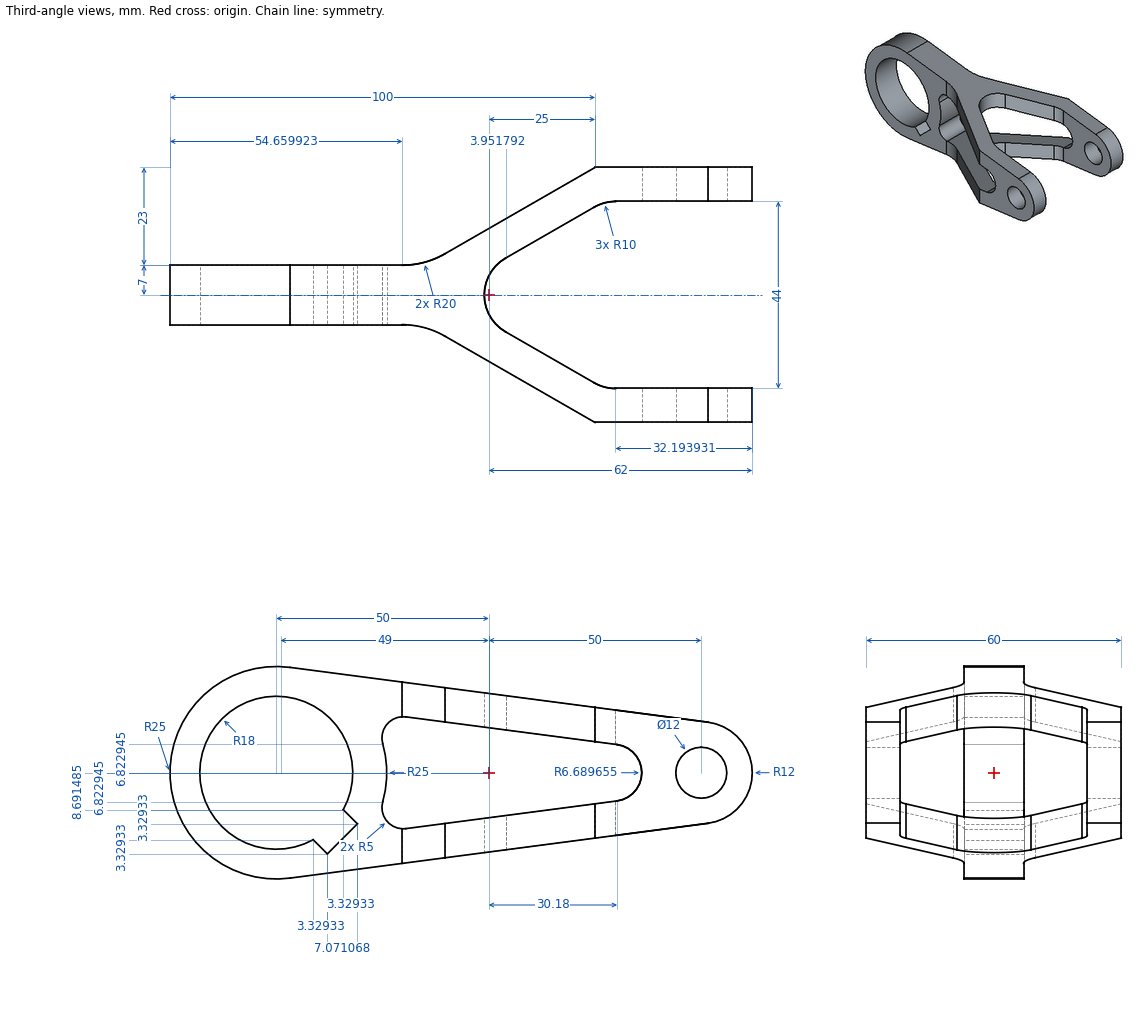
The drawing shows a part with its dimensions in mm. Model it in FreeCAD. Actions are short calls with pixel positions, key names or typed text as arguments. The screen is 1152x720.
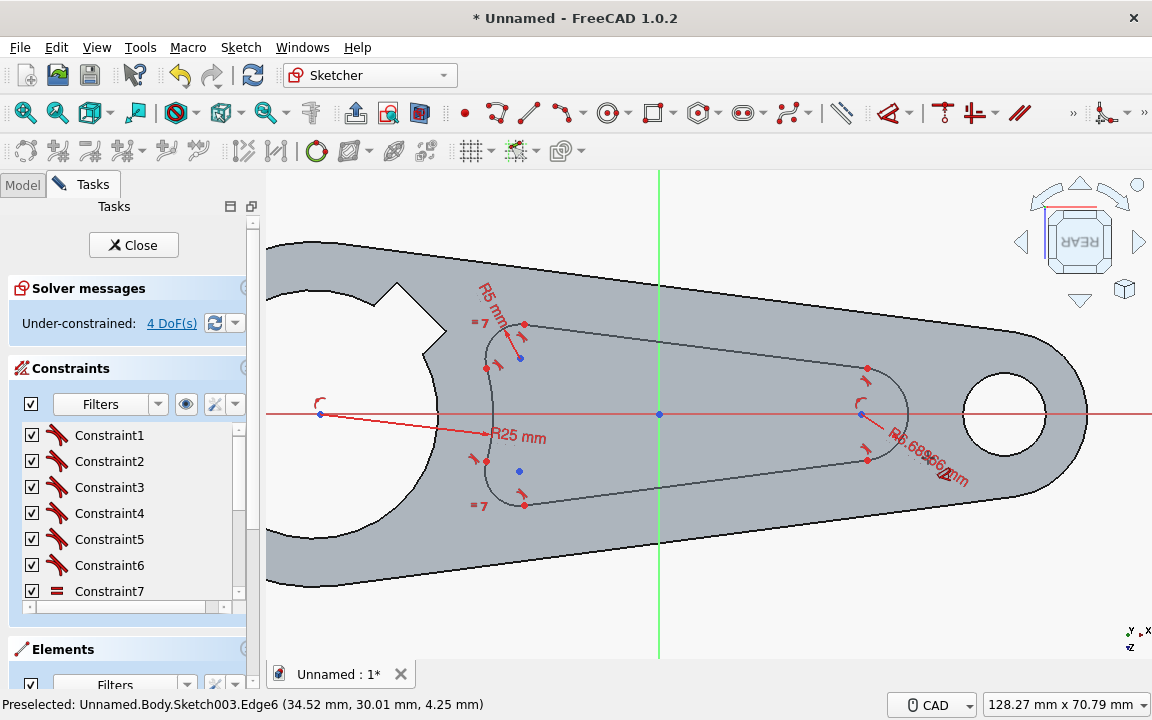
click(320, 414)
click(412, 448)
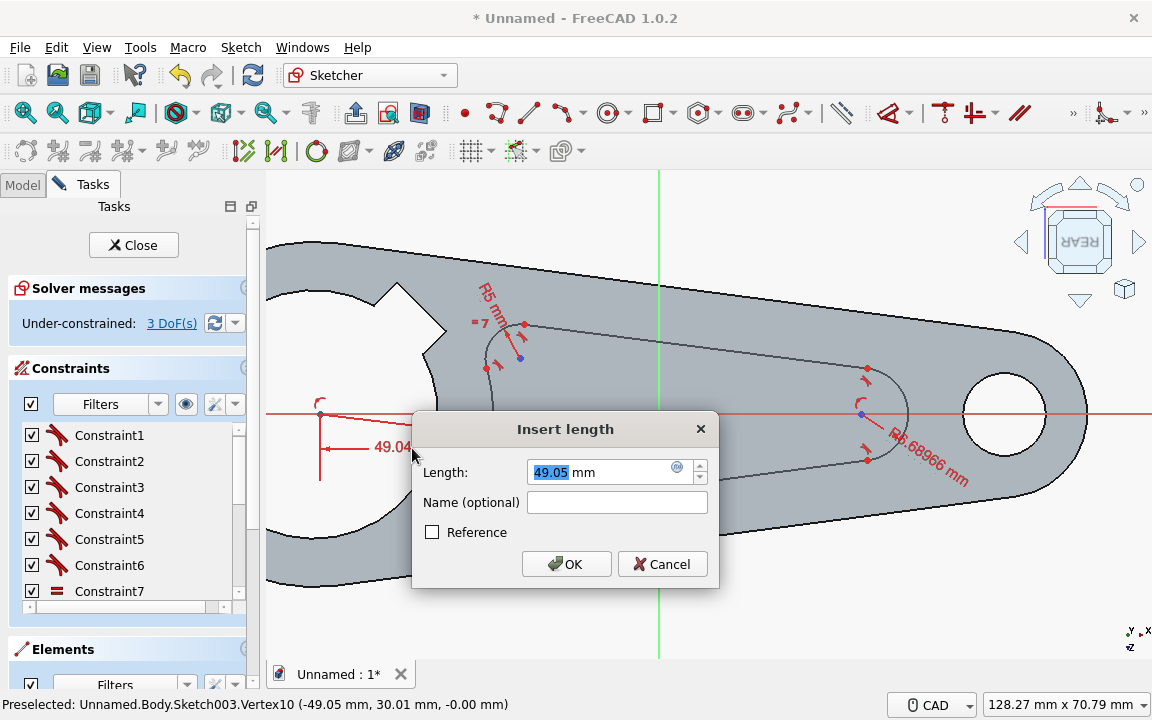
text(49)
key(Return)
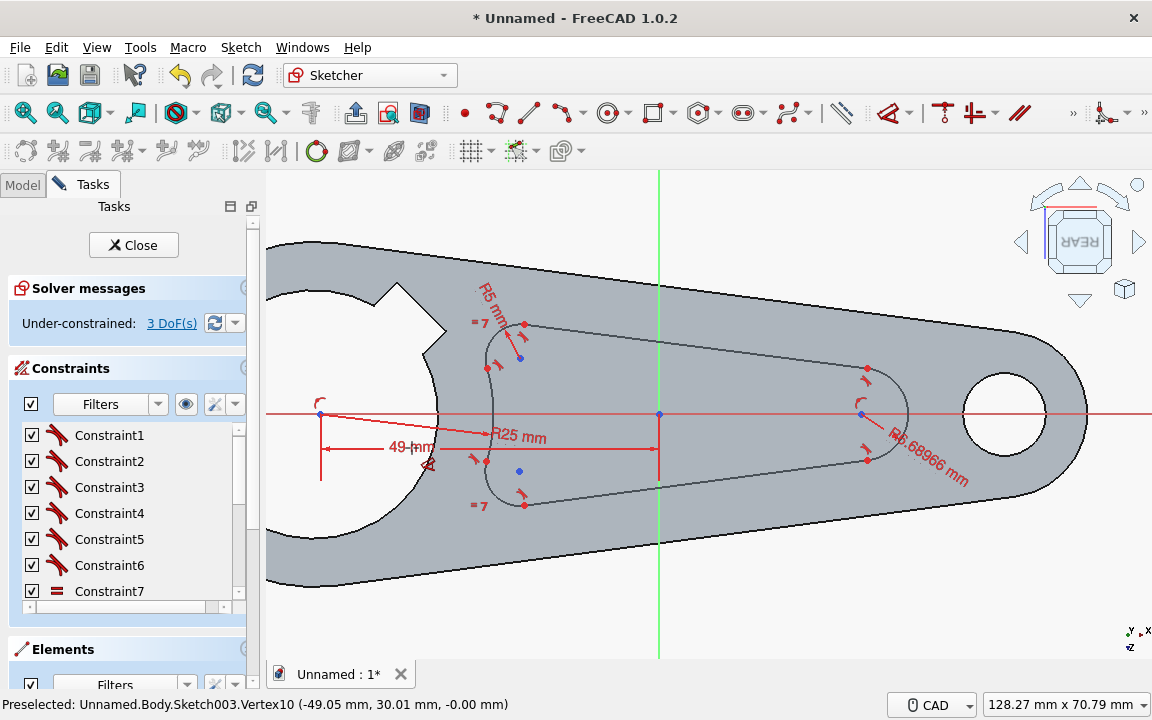
click(868, 369)
click(763, 335)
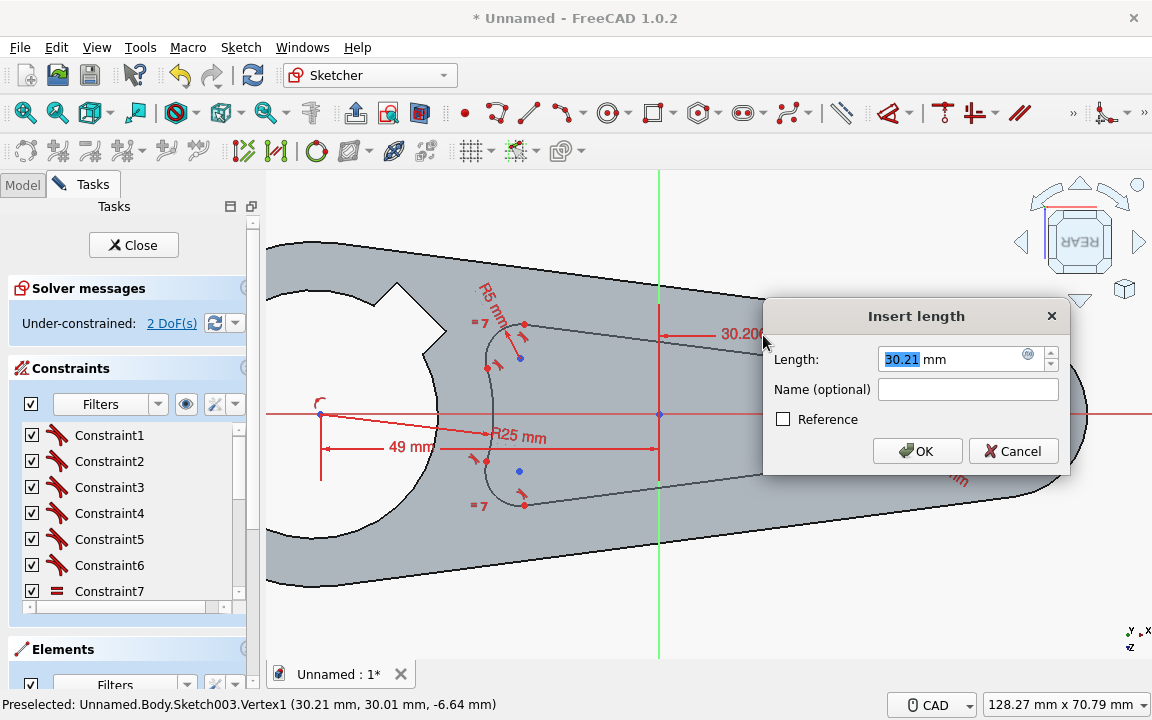
text(30.18)
key(Return)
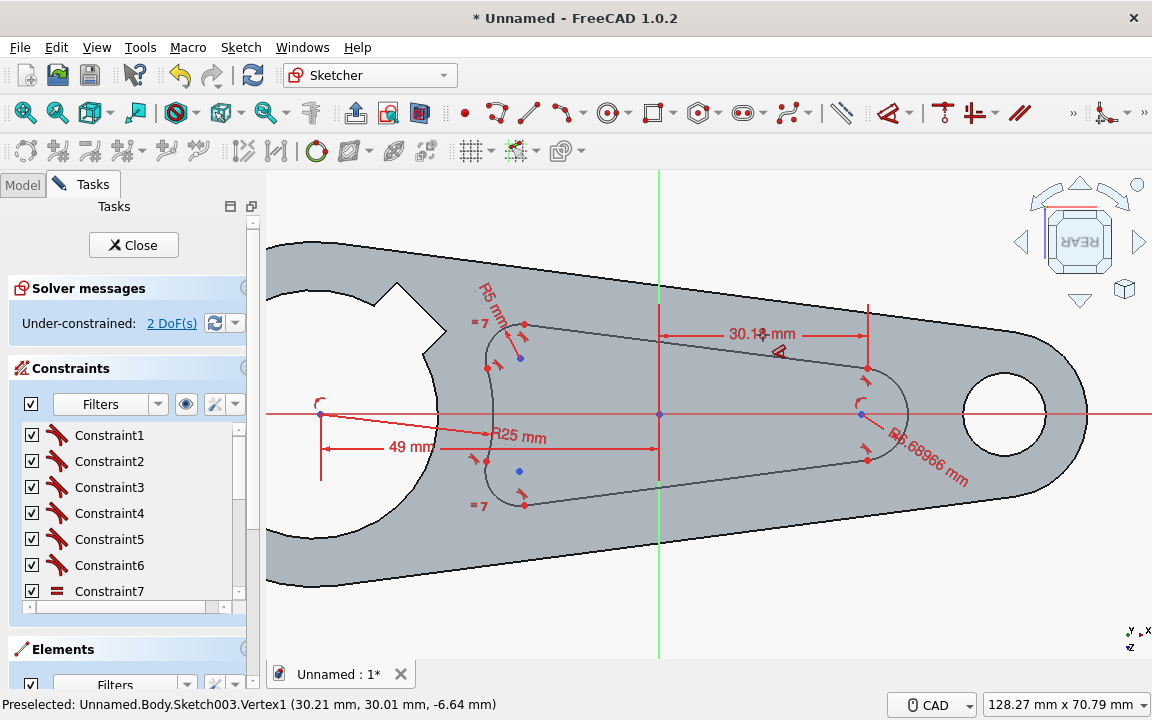
click(487, 368)
click(453, 391)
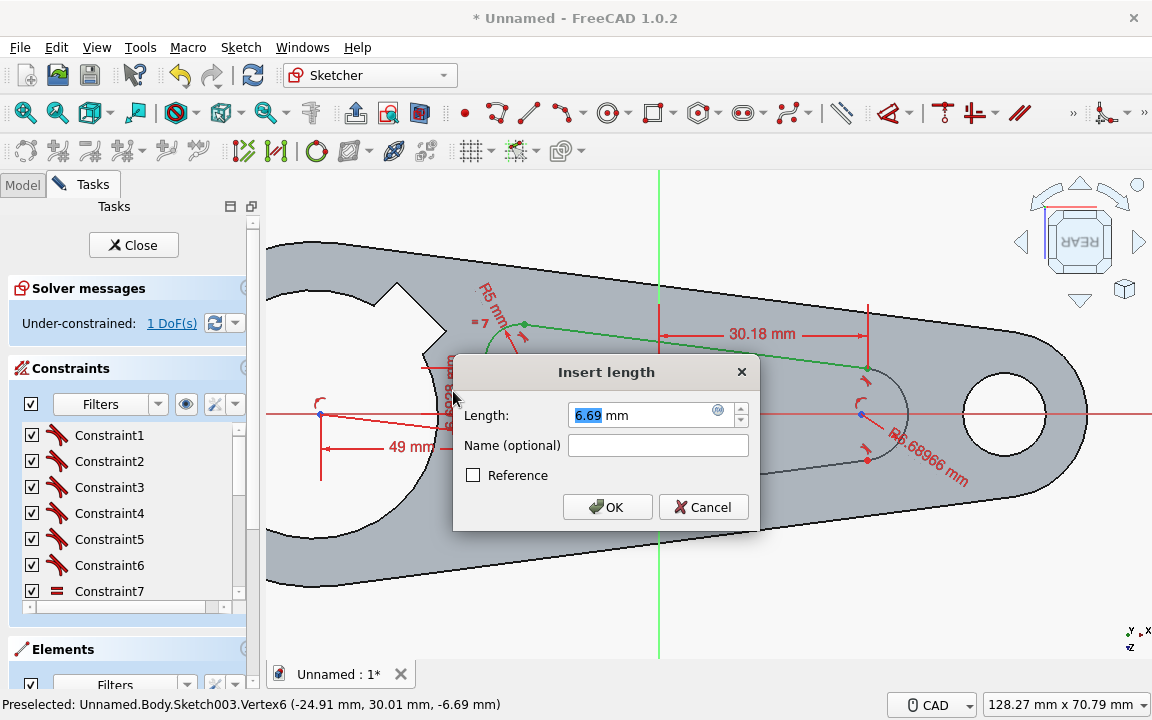
text(6.822945)
key(Return)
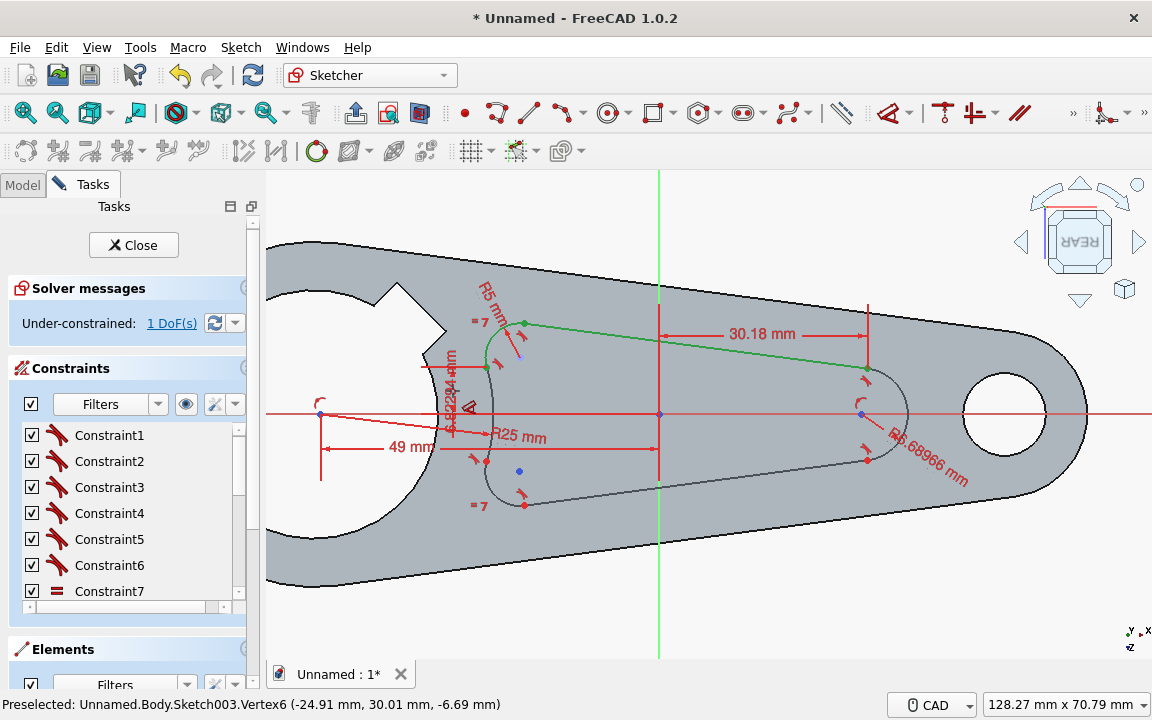
click(487, 462)
click(693, 438)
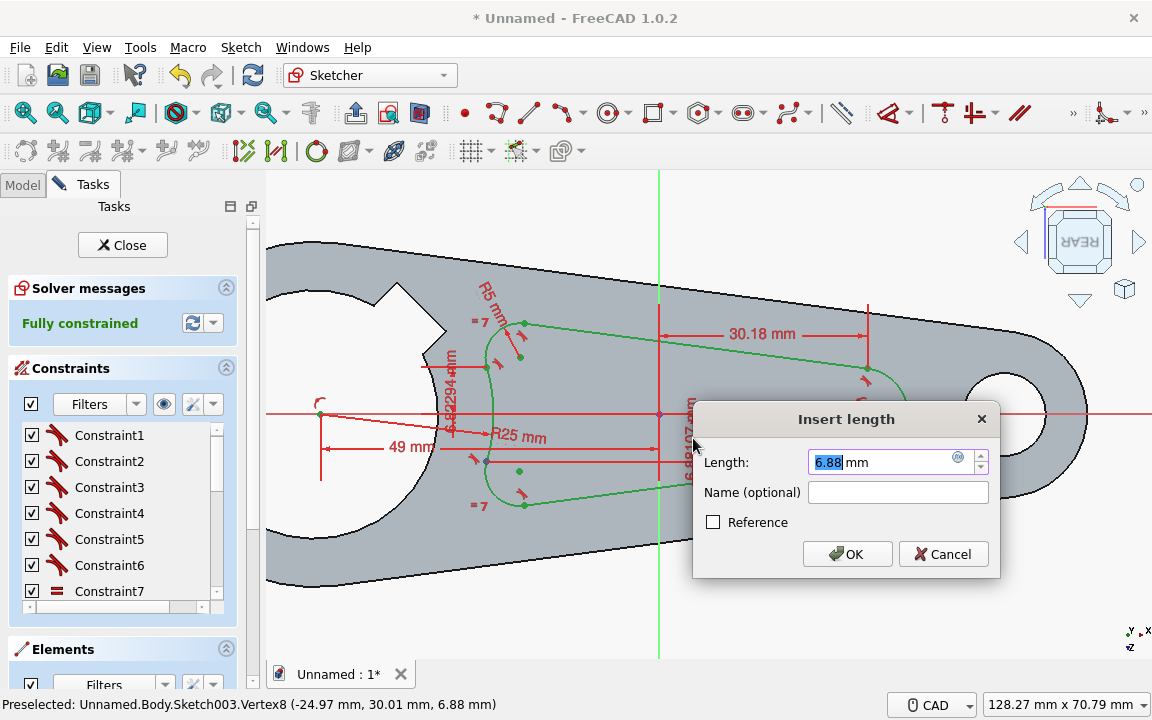
text(6.822945)
key(Return)
key(Escape)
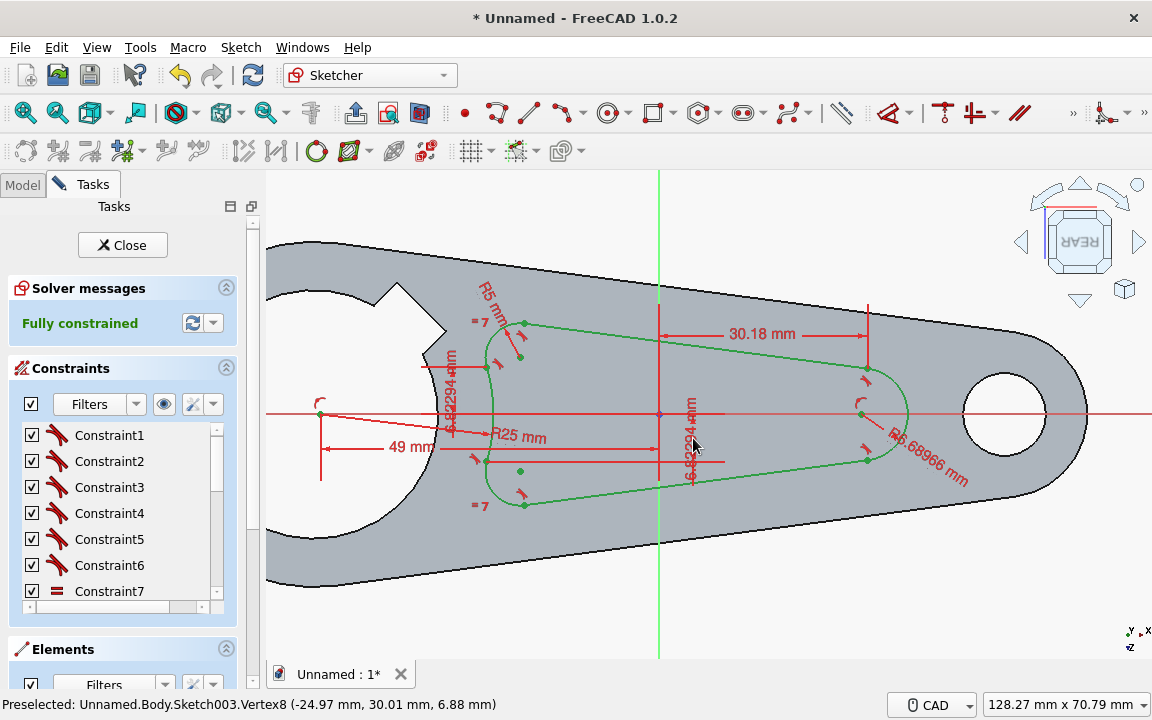
click(123, 245)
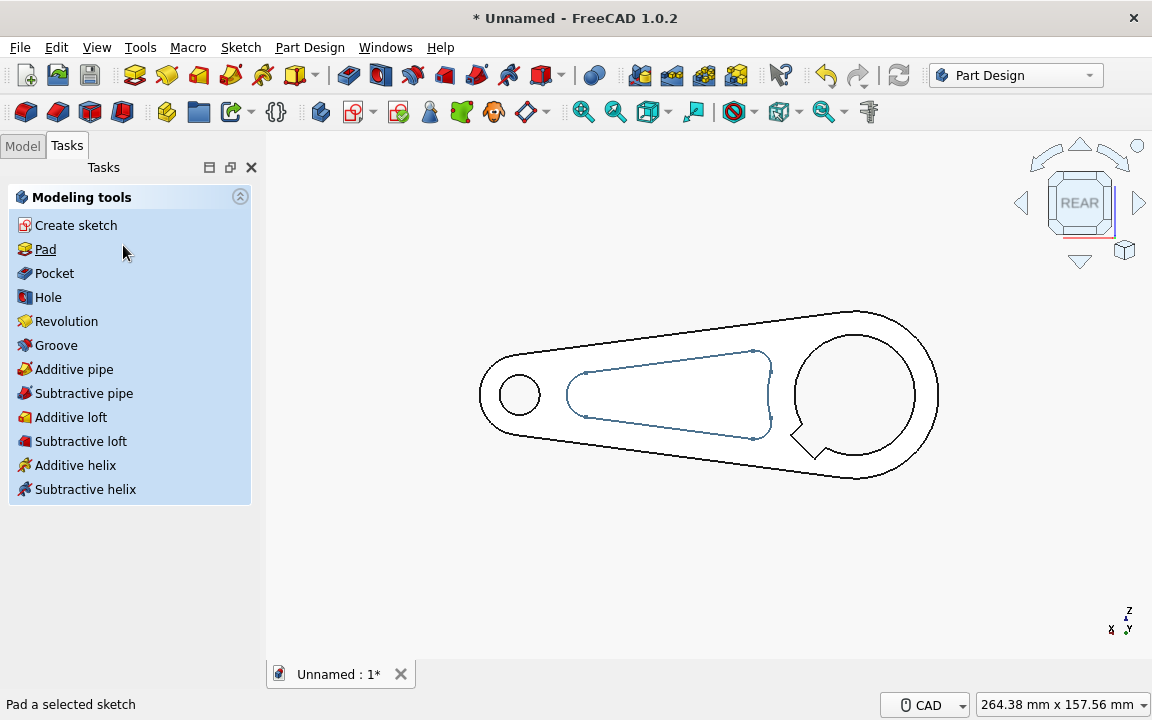
click(350, 76)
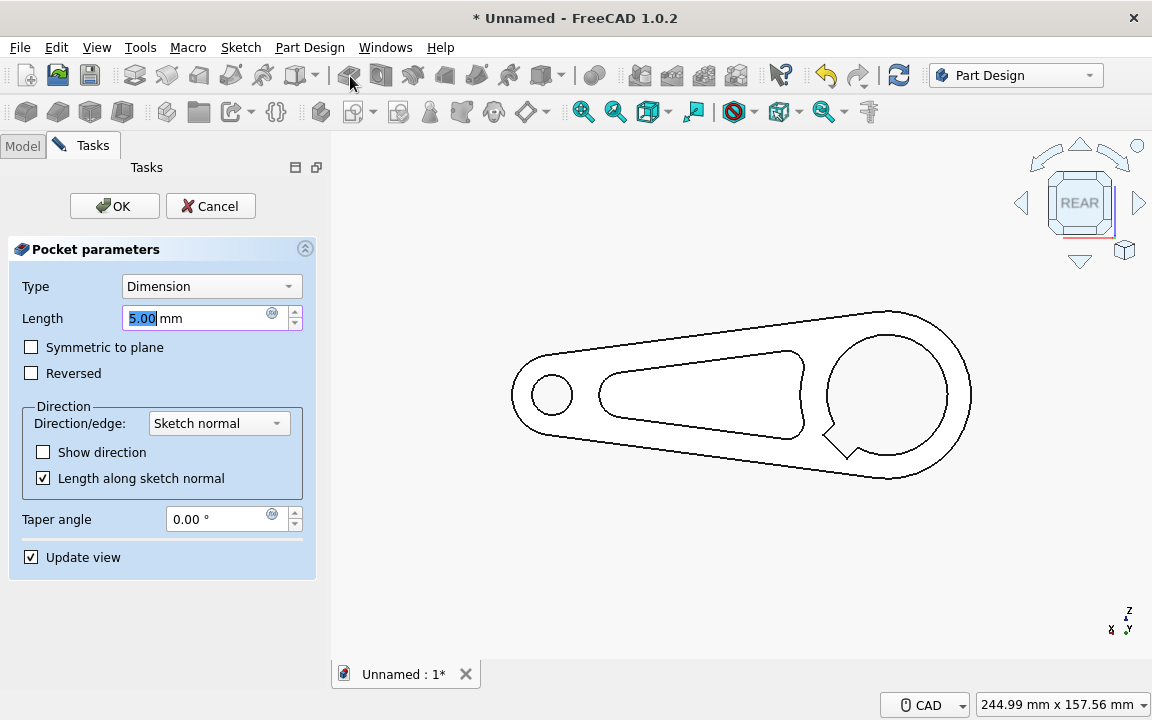
click(212, 286)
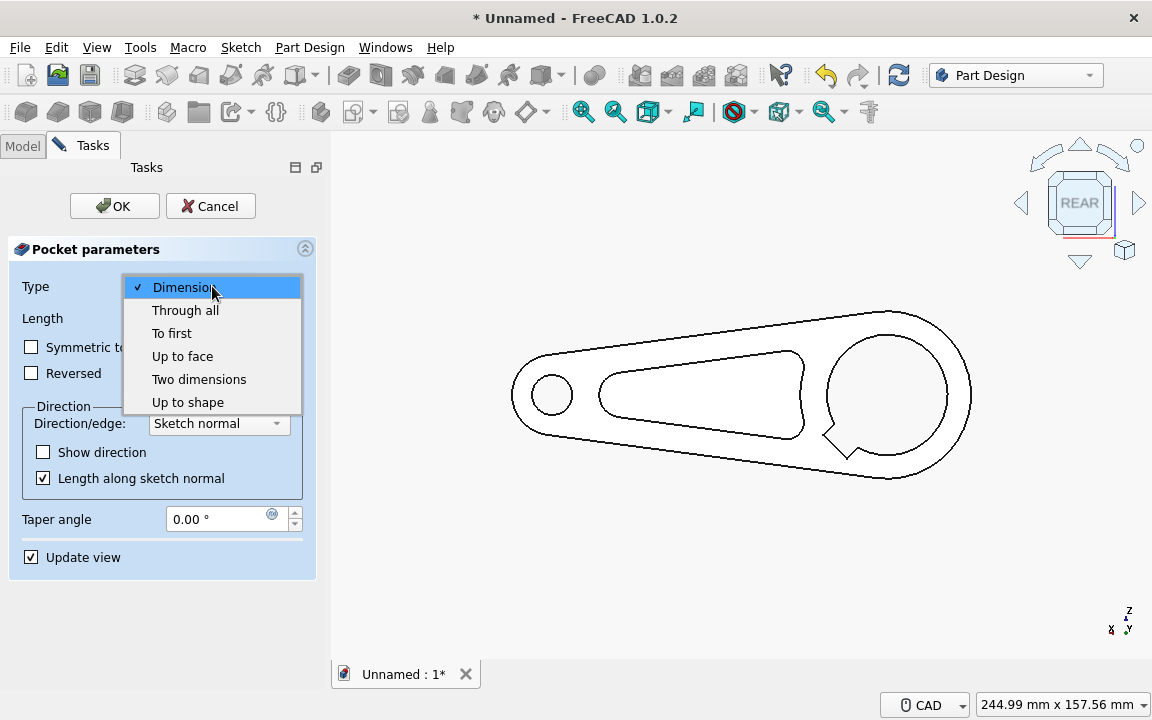
click(212, 310)